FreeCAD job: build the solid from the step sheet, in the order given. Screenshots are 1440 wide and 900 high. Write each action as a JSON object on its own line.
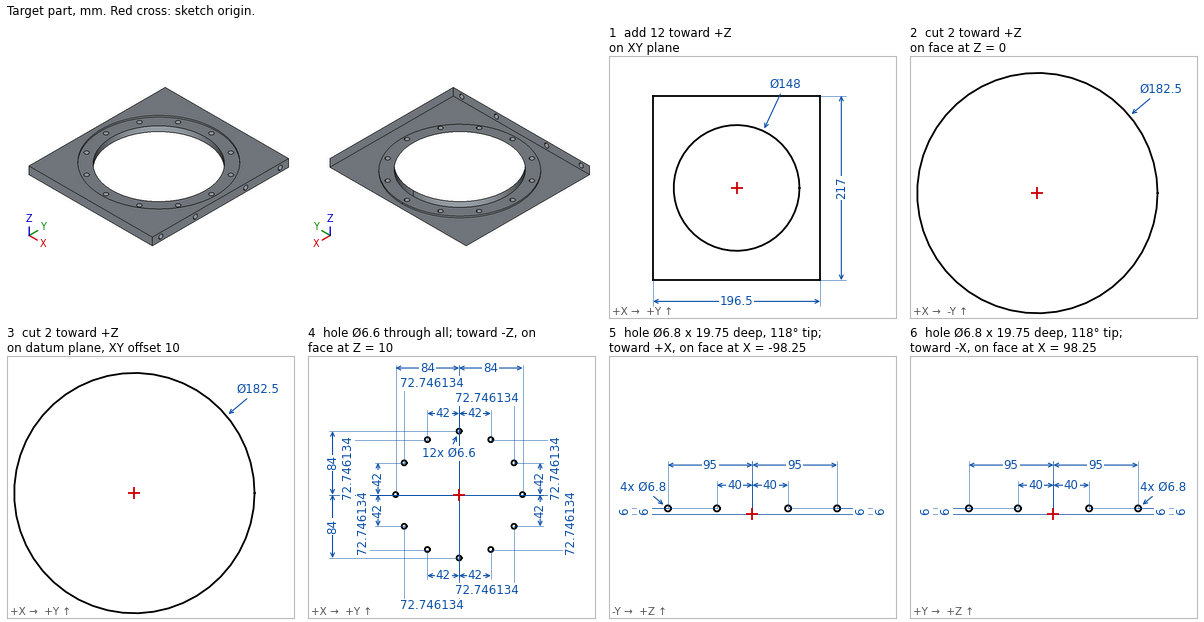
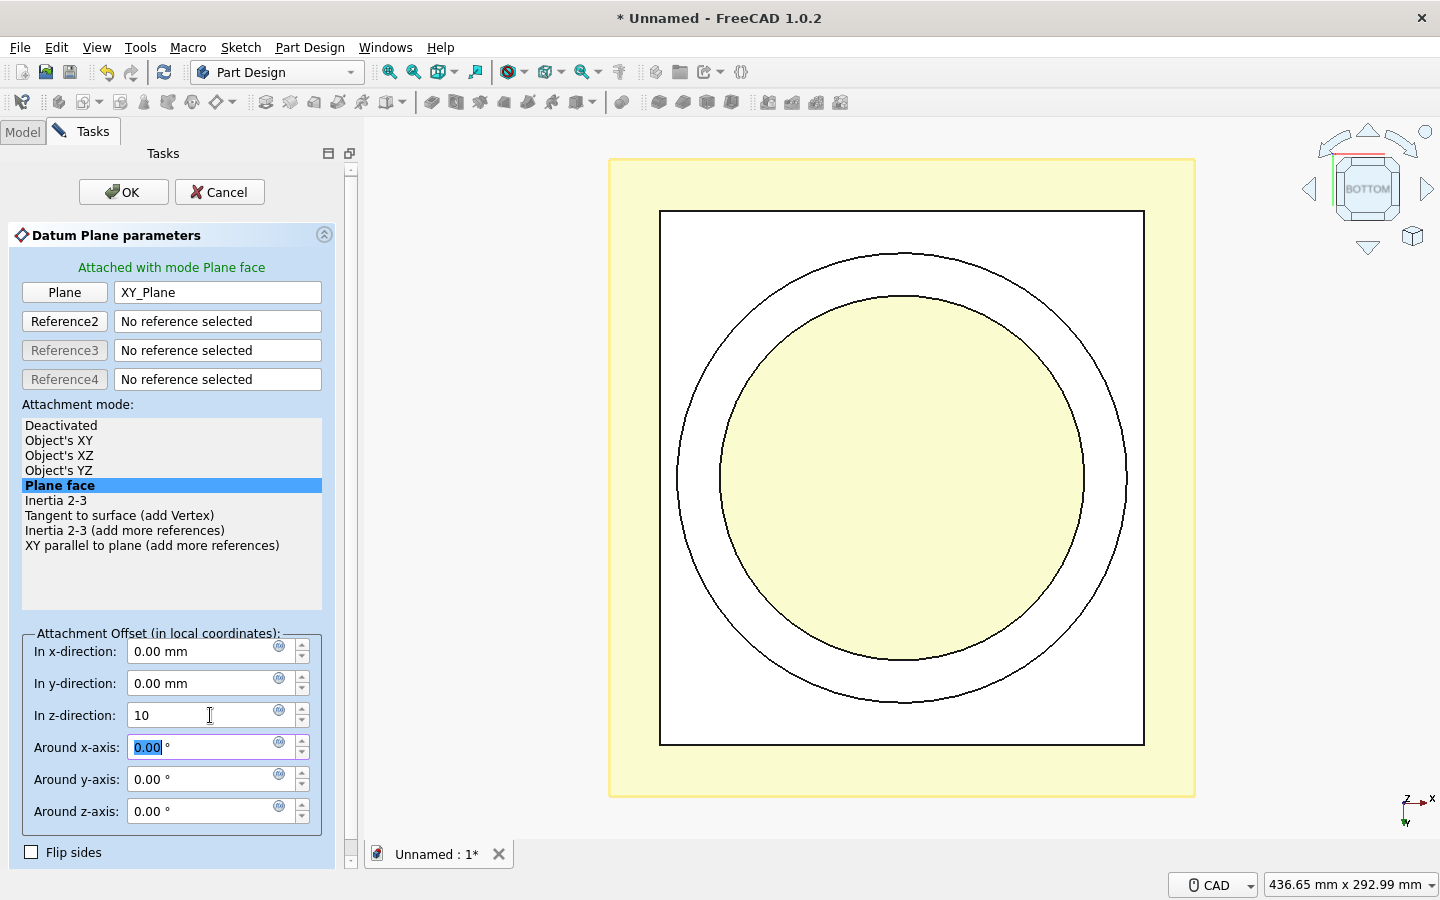
{"action": "left_click", "coordinate": [124, 192]}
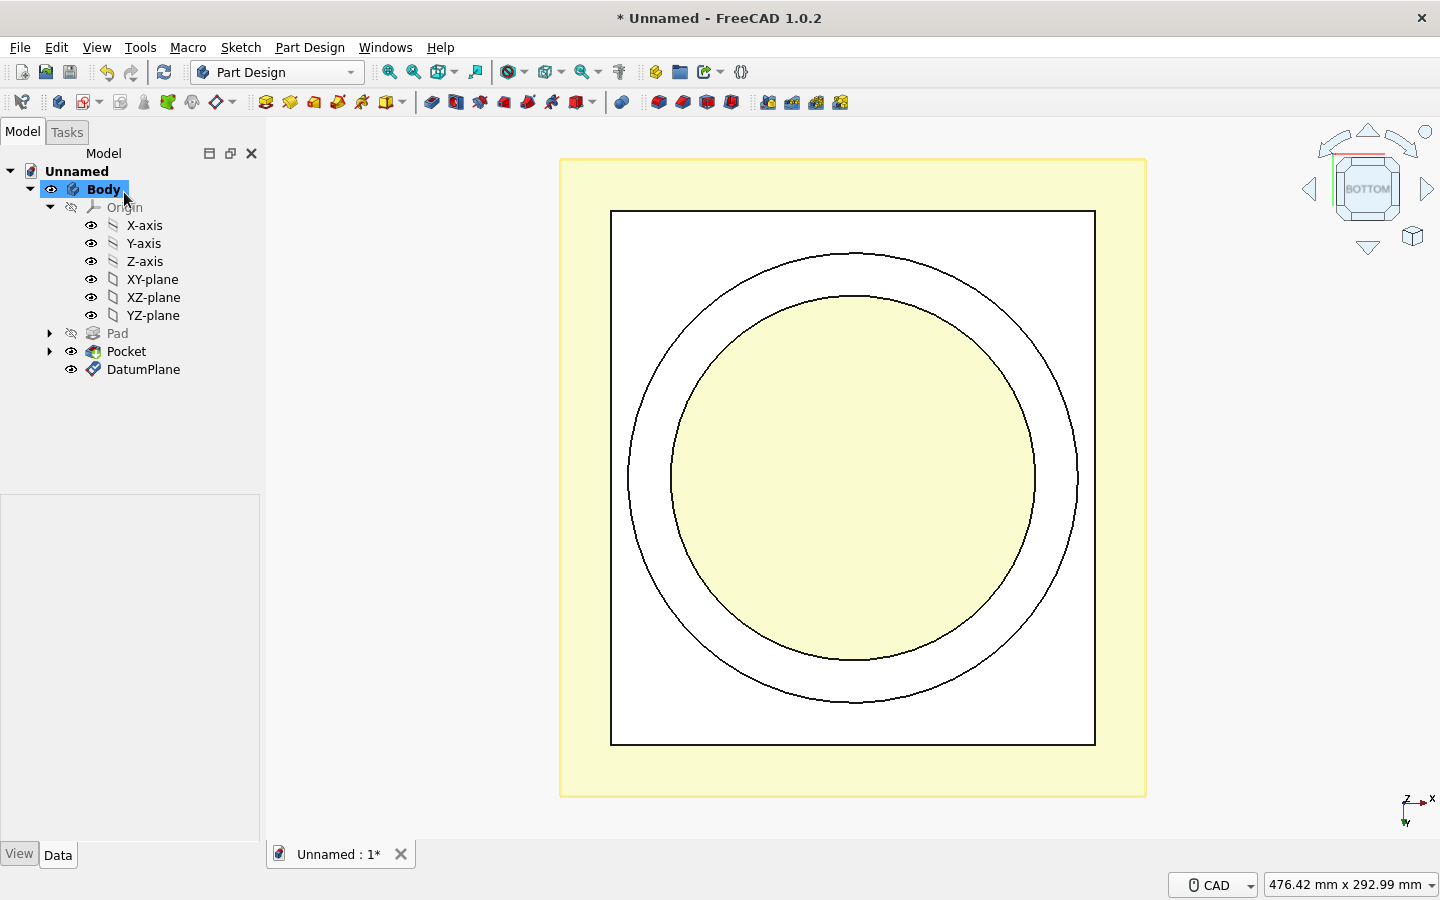
{"action": "left_click", "coordinate": [116, 369]}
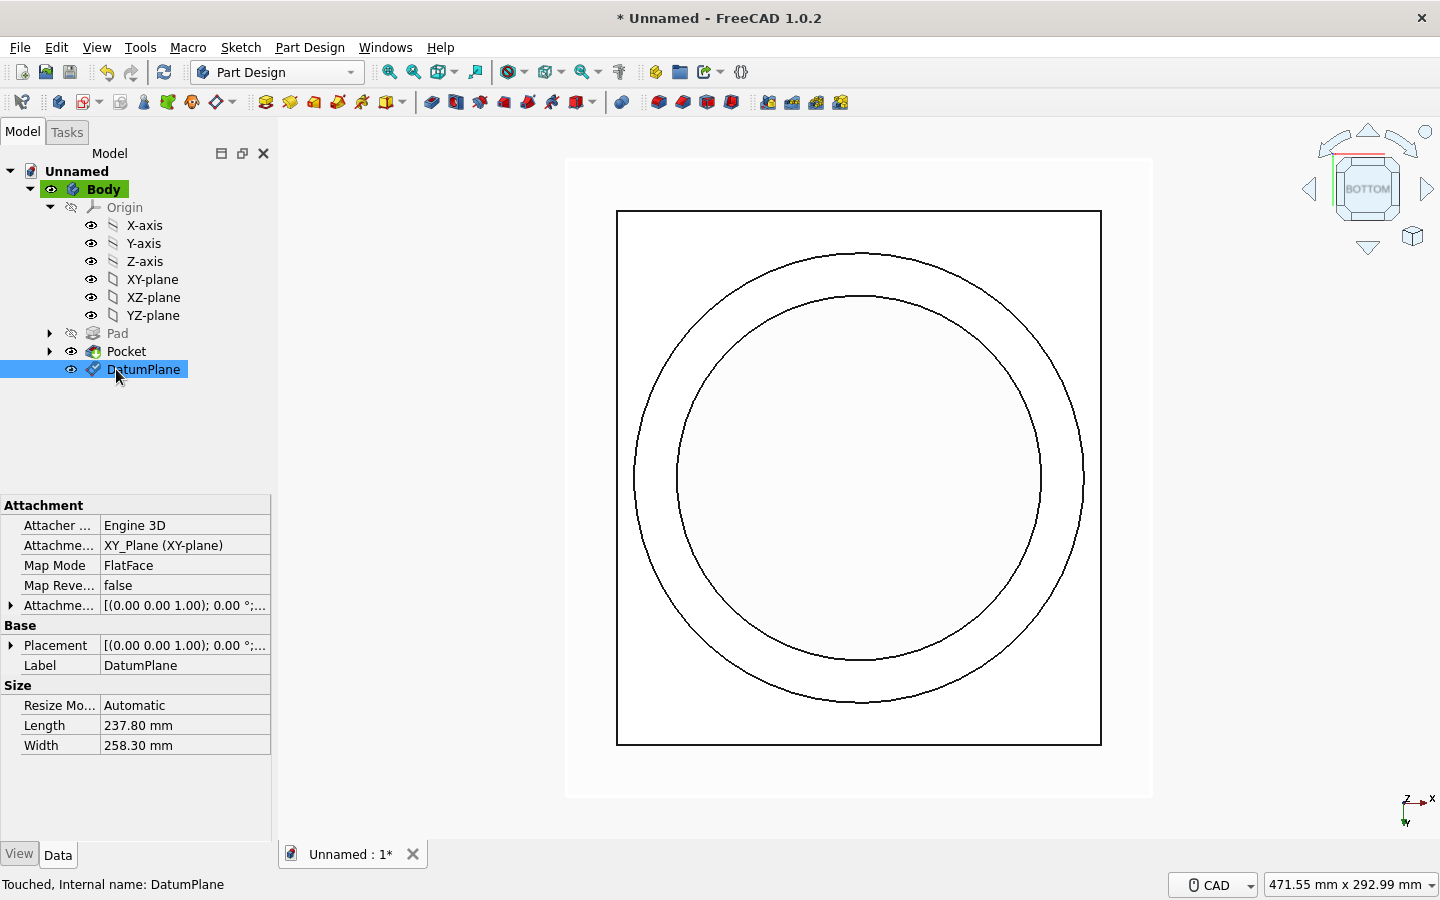
{"action": "left_click", "coordinate": [84, 102]}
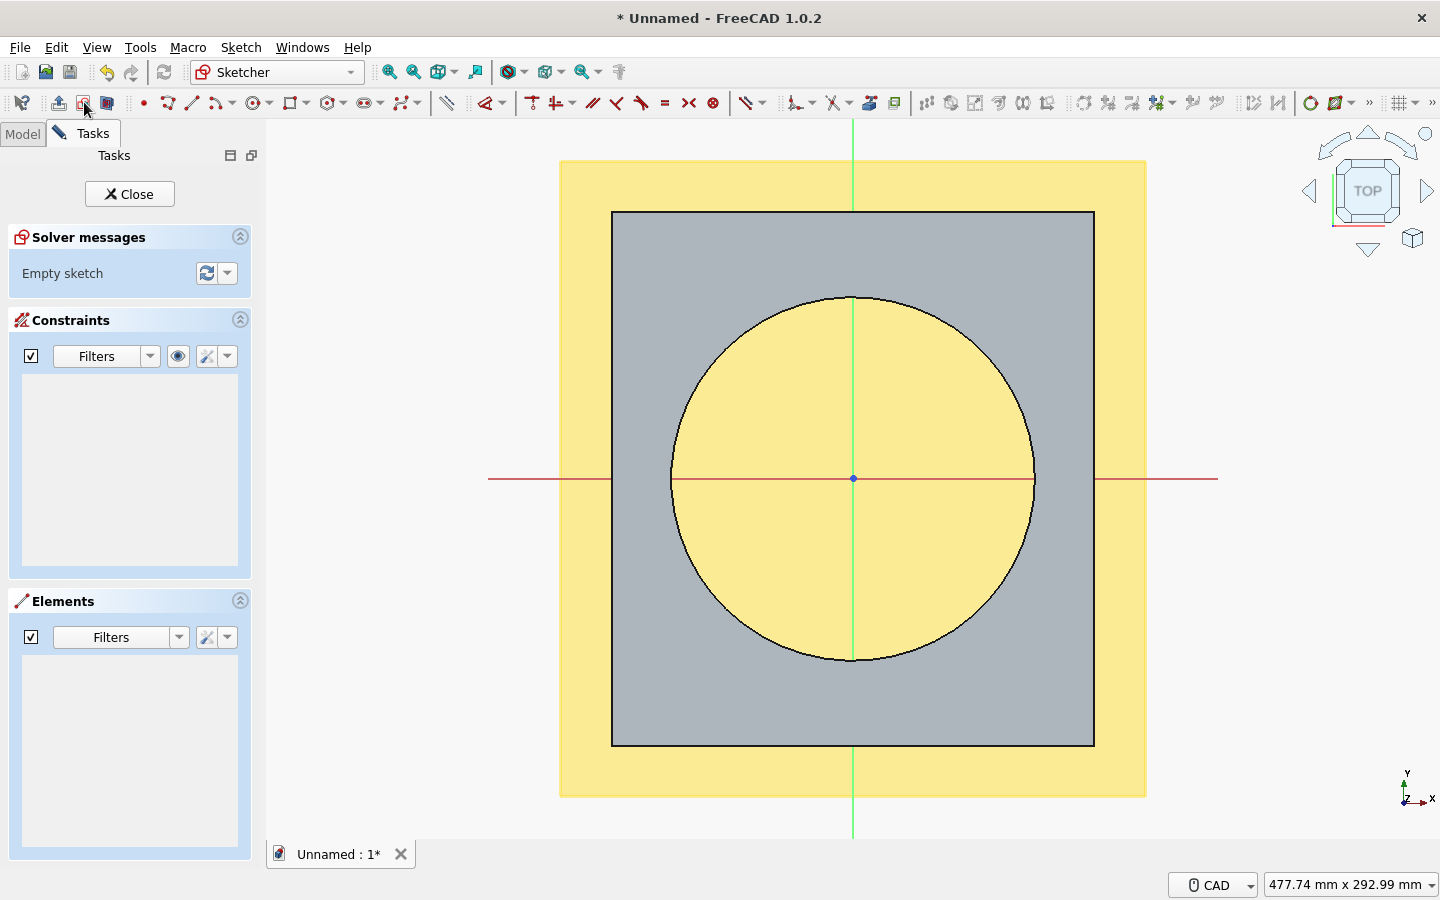
{"action": "left_click", "coordinate": [108, 104]}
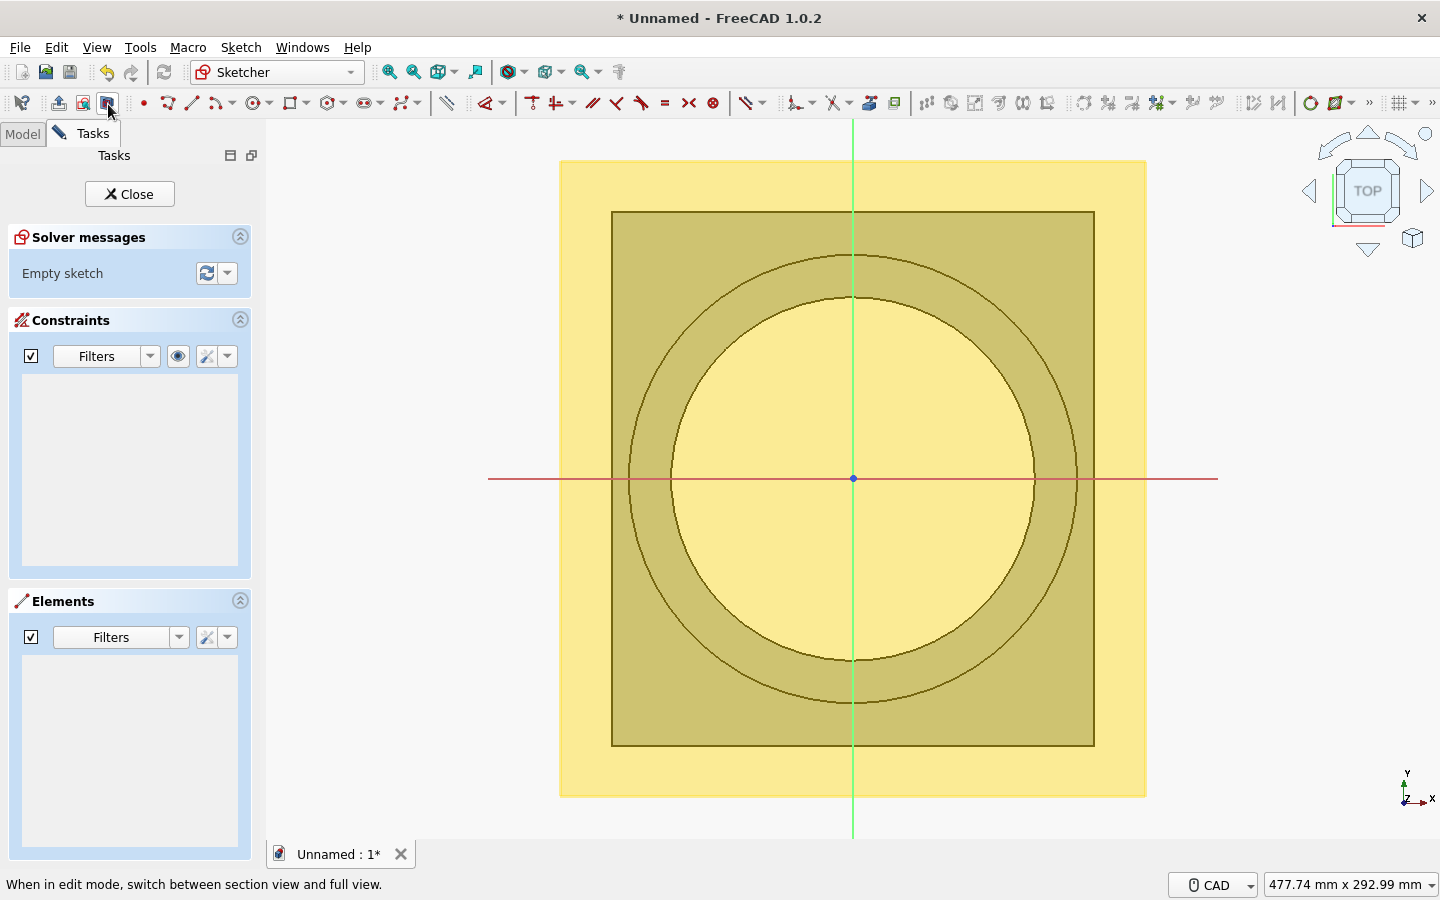
{"action": "left_click", "coordinate": [254, 104]}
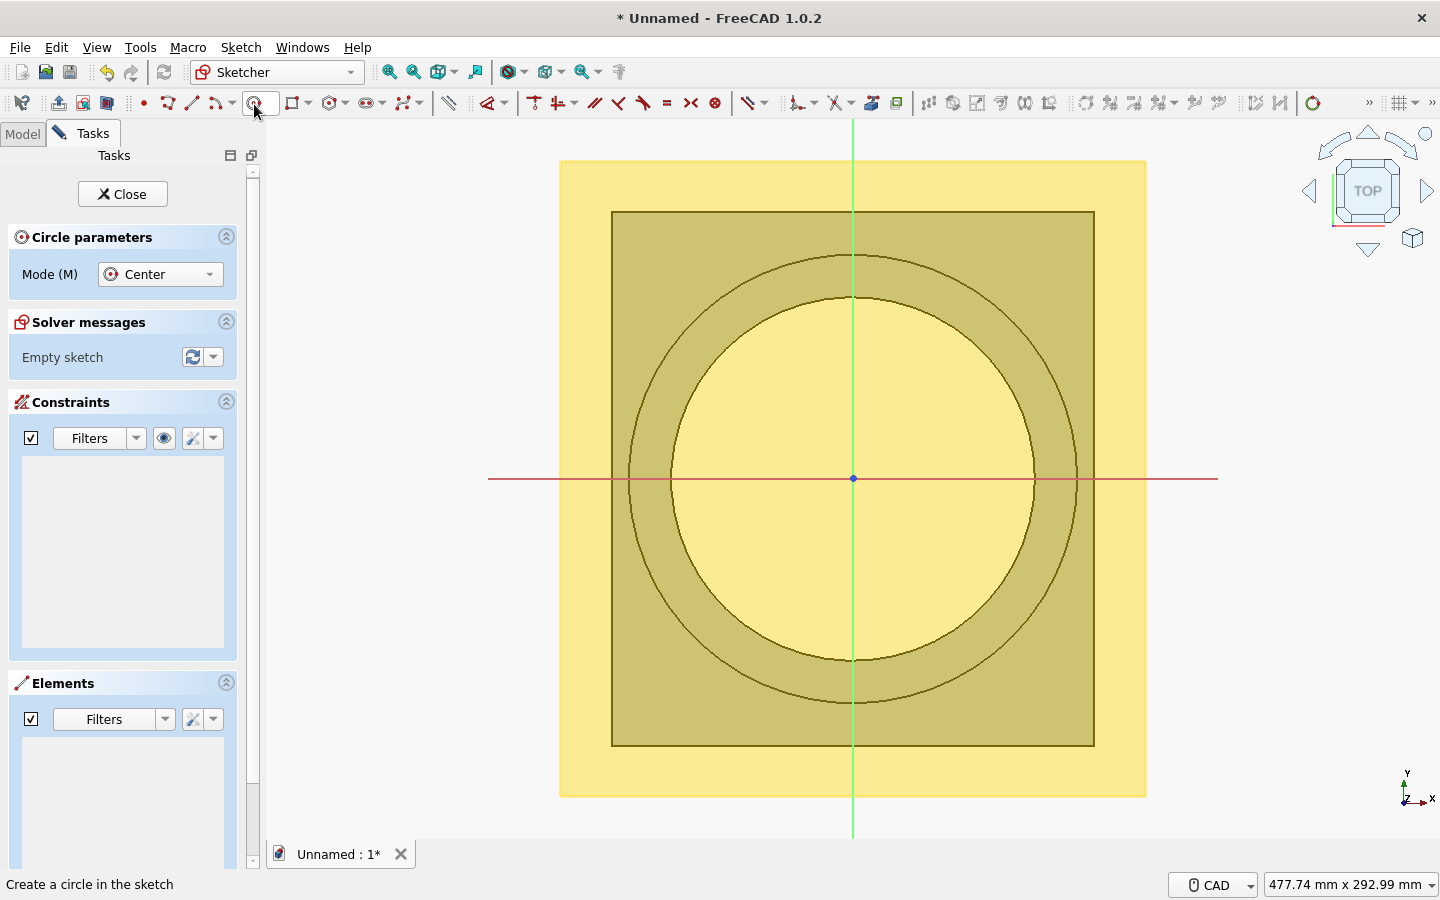
{"action": "left_click", "coordinate": [853, 479]}
{"action": "mouse_move", "coordinate": [1012, 320]}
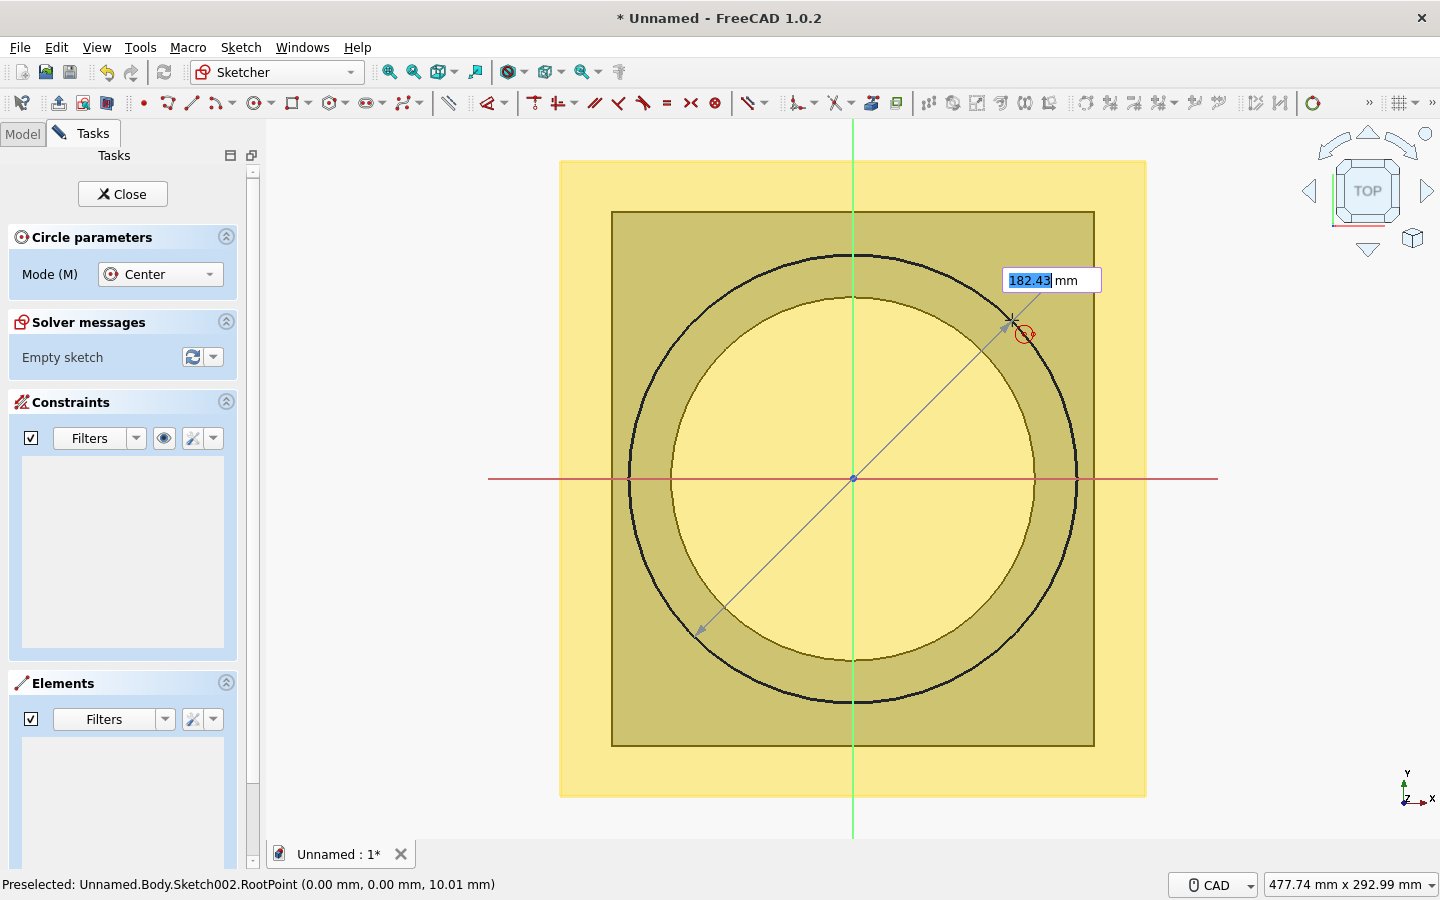
{"action": "type", "text": "182.5"}
{"action": "key", "text": "Return"}
{"action": "key", "text": "Escape"}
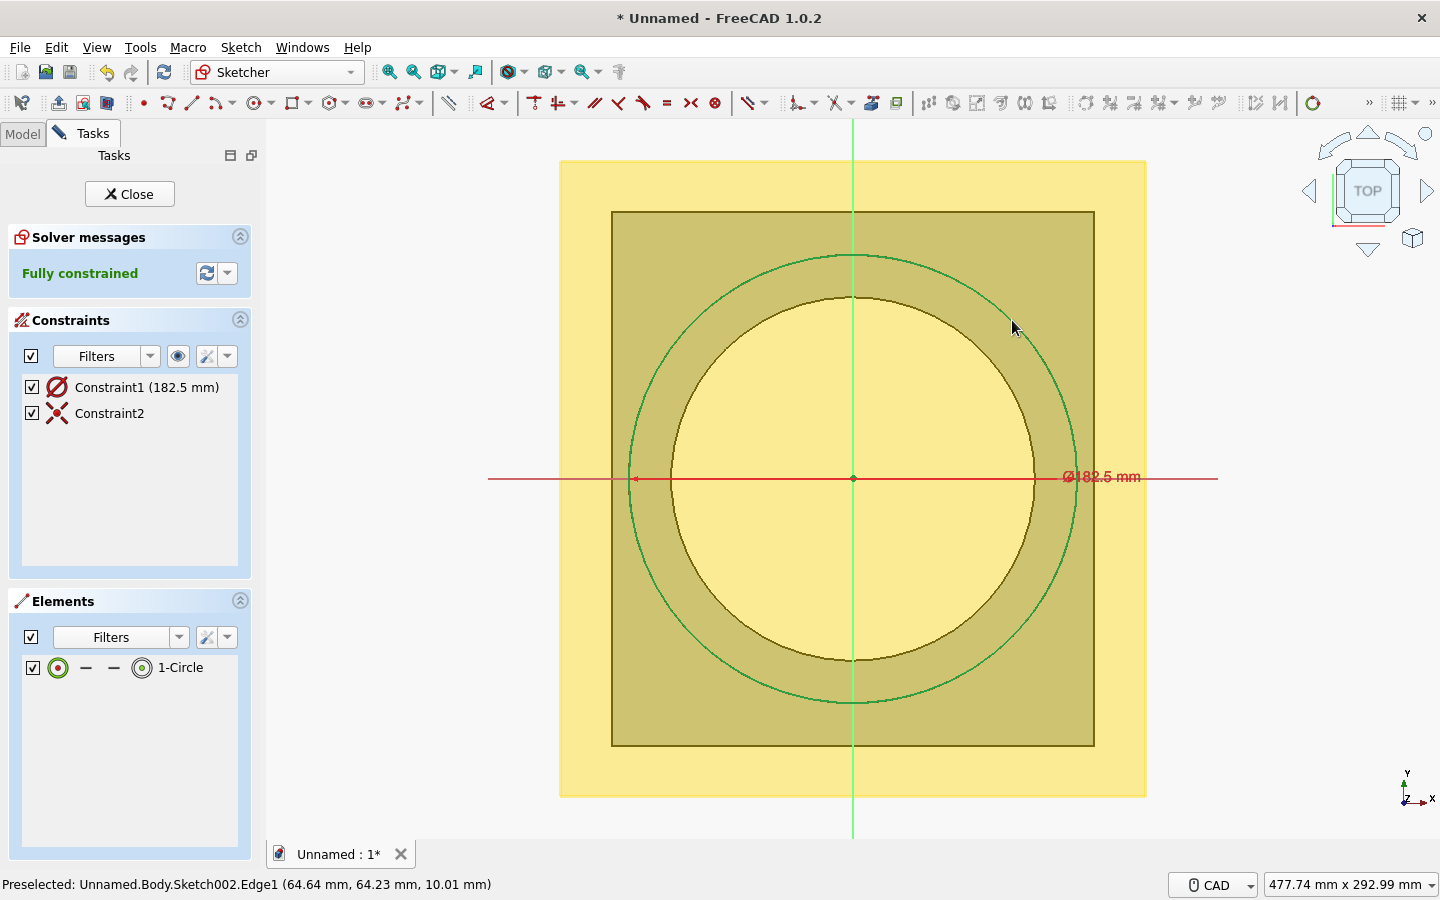
{"action": "left_click", "coordinate": [130, 194]}